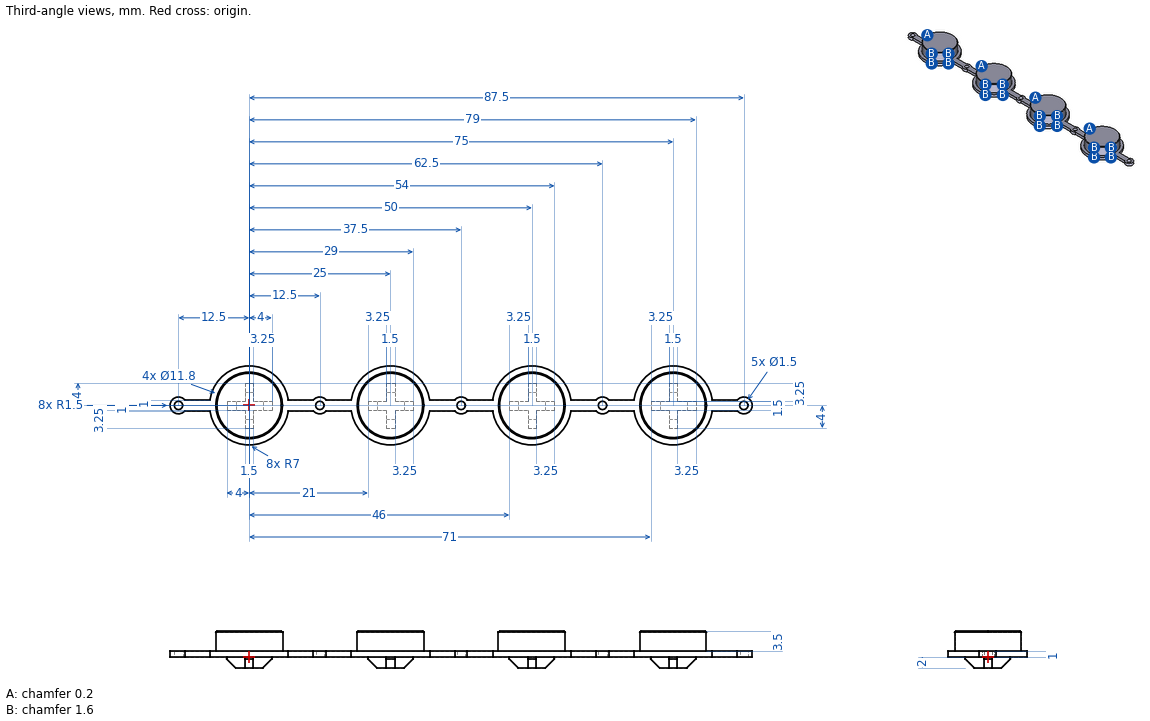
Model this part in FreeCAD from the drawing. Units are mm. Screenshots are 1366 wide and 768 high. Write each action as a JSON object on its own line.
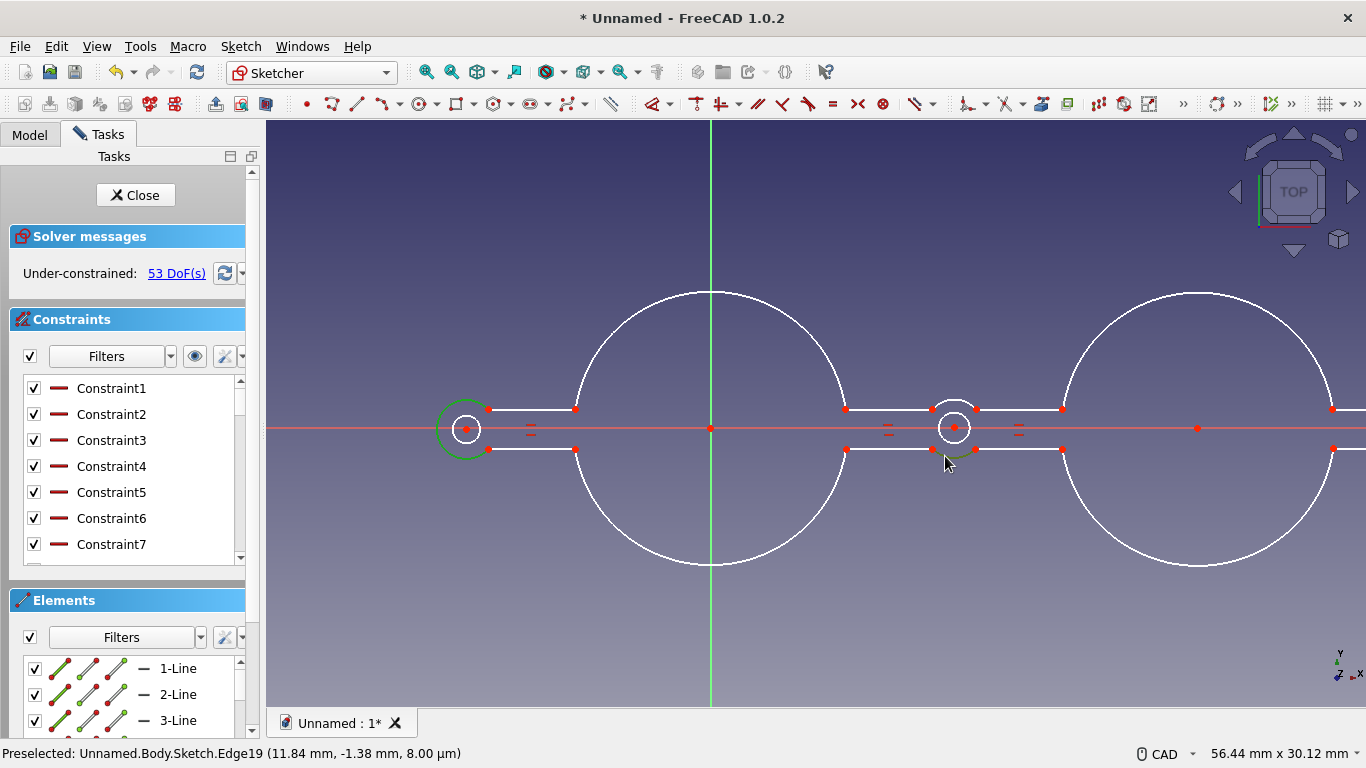
{"action": "scroll", "coordinate": [448, 407], "scroll_direction": "down", "scroll_amount": 6}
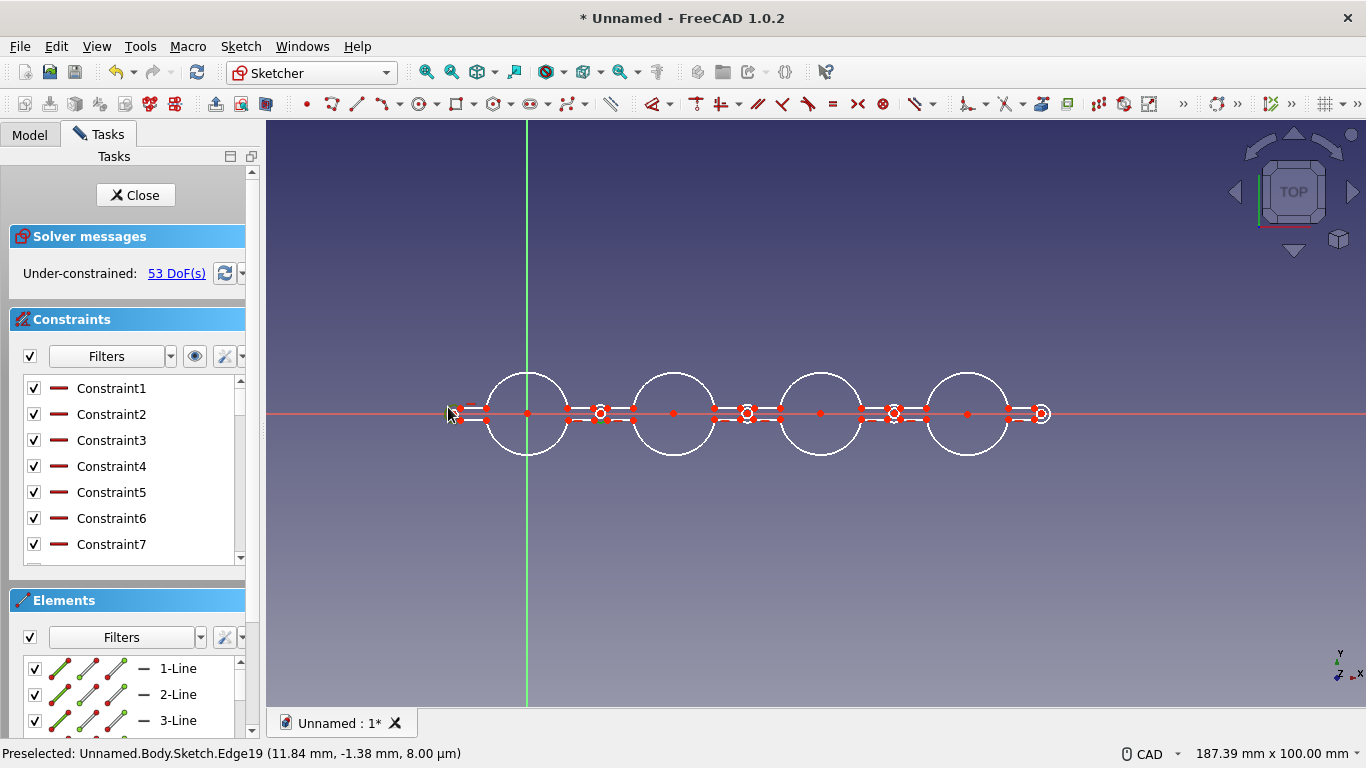
{"action": "scroll", "coordinate": [744, 422], "scroll_direction": "up", "scroll_amount": 6}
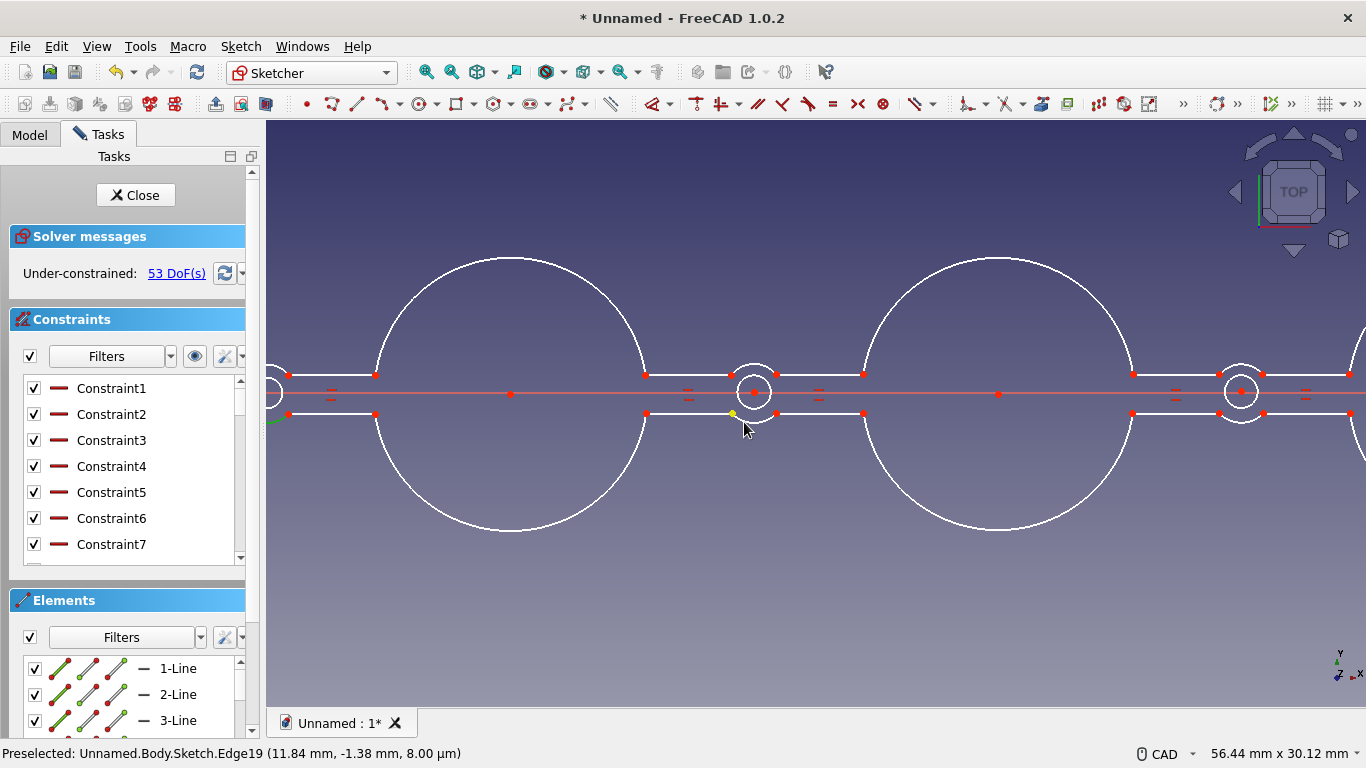
{"action": "left_click", "coordinate": [745, 421]}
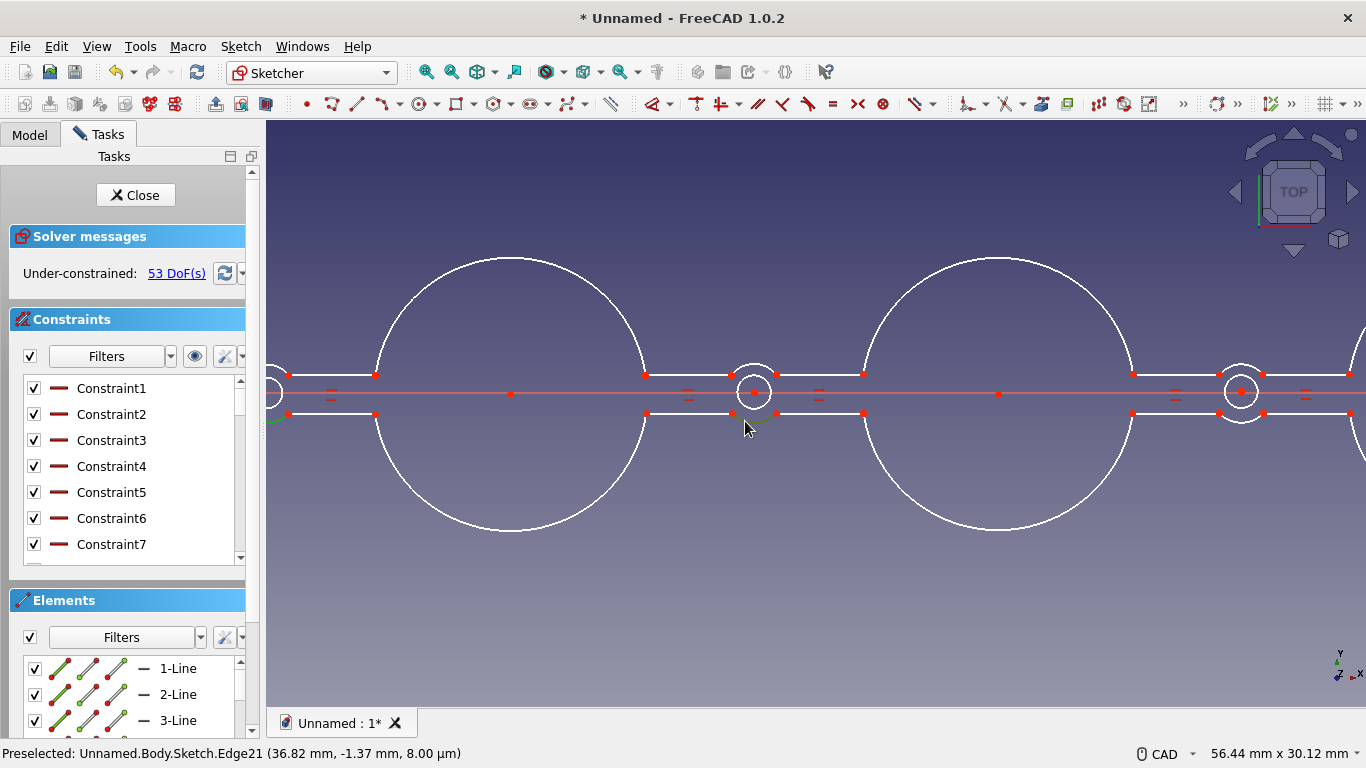
{"action": "scroll", "coordinate": [745, 422], "scroll_direction": "down", "scroll_amount": 6}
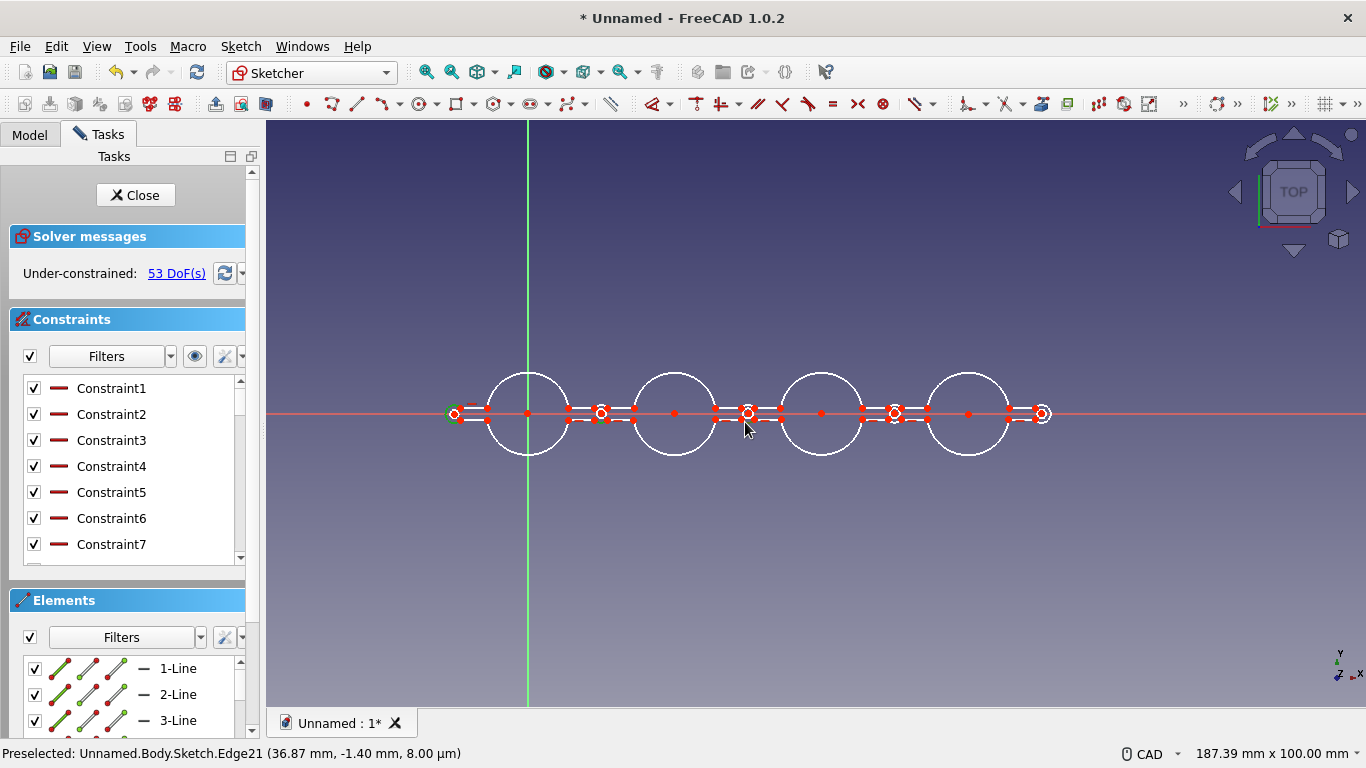
{"action": "scroll", "coordinate": [892, 422], "scroll_direction": "up", "scroll_amount": 6}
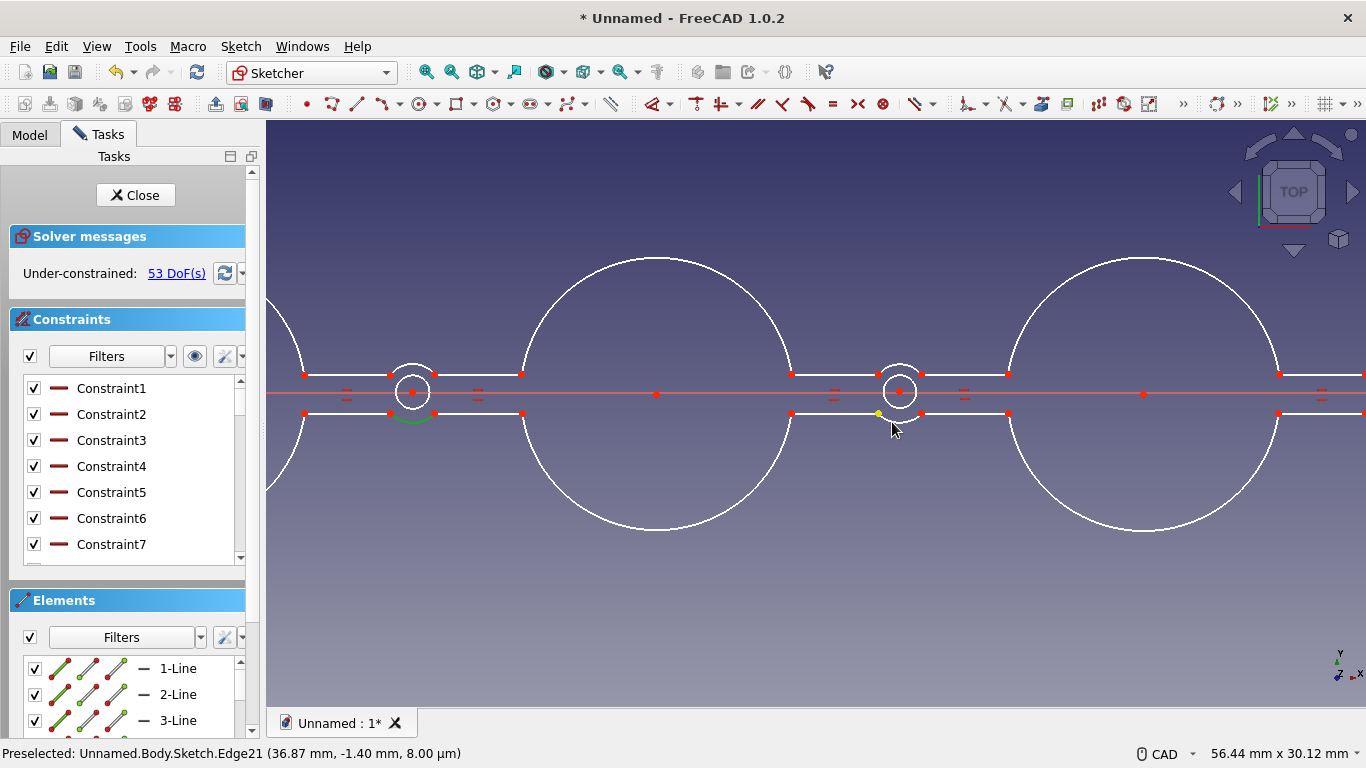
{"action": "left_click", "coordinate": [891, 421]}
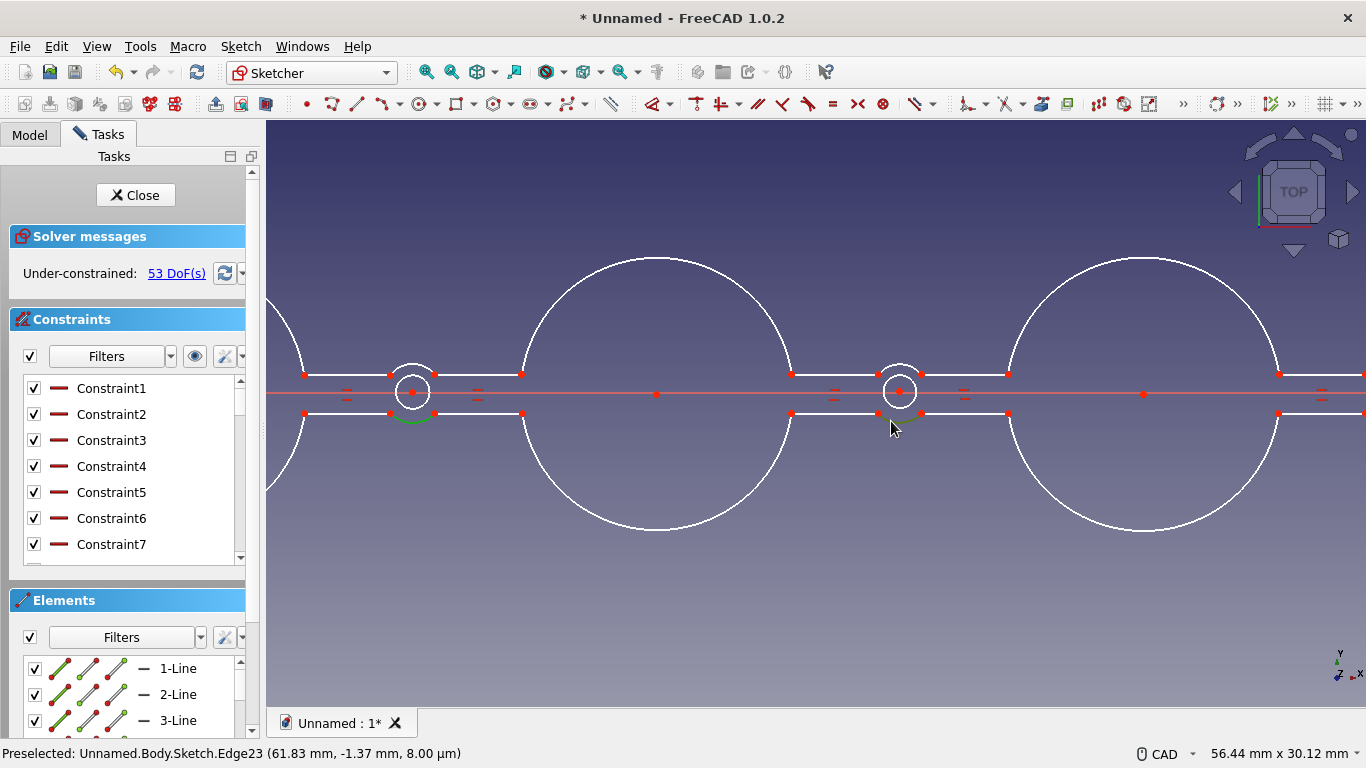
{"action": "scroll", "coordinate": [892, 422], "scroll_direction": "down", "scroll_amount": 6}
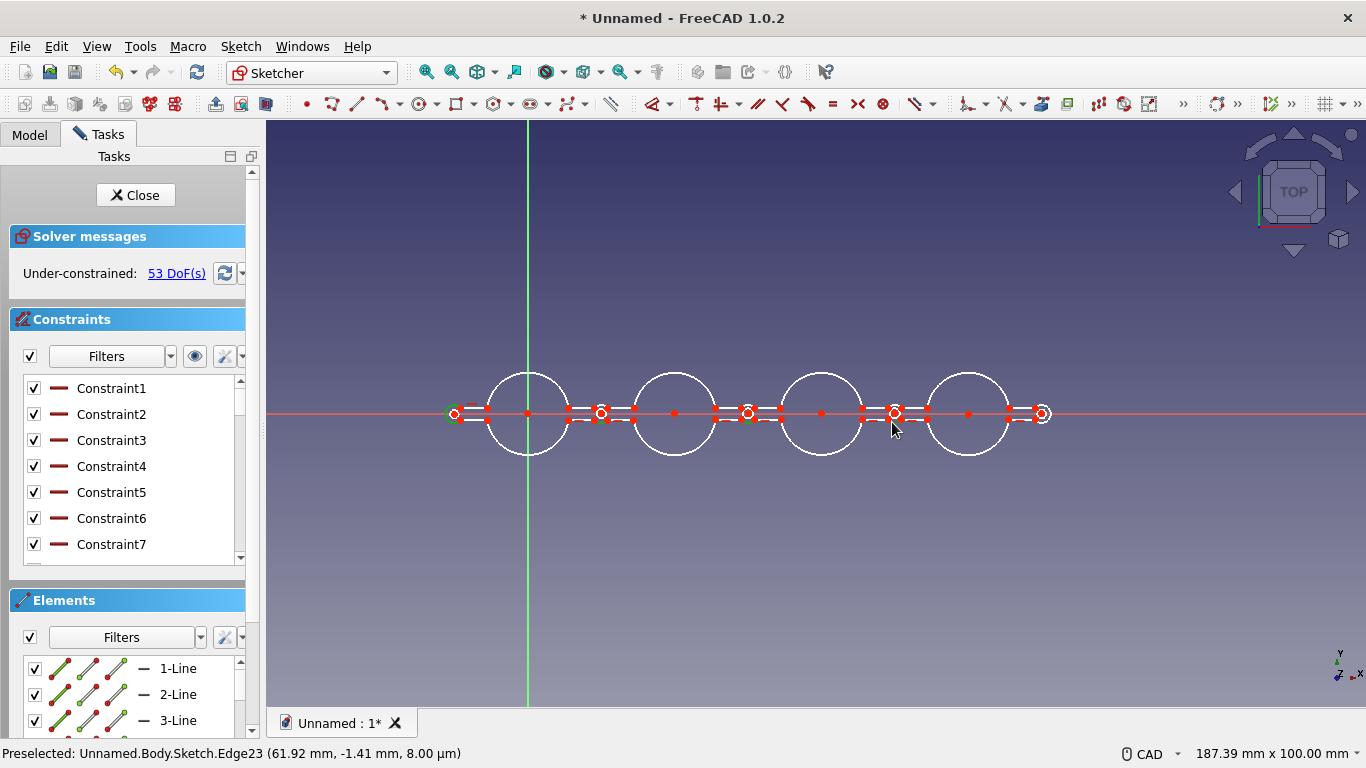
{"action": "scroll", "coordinate": [1047, 421], "scroll_direction": "up", "scroll_amount": 6}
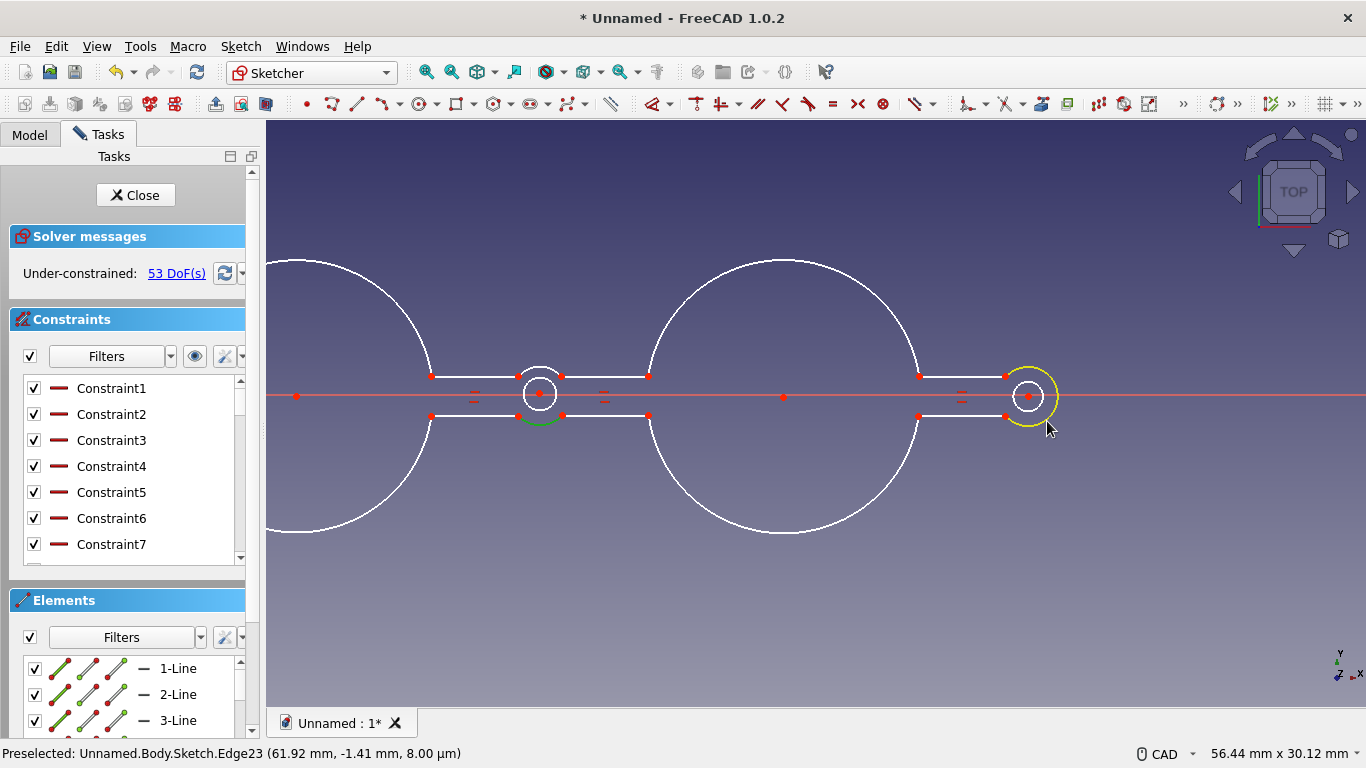
{"action": "left_click", "coordinate": [1045, 421]}